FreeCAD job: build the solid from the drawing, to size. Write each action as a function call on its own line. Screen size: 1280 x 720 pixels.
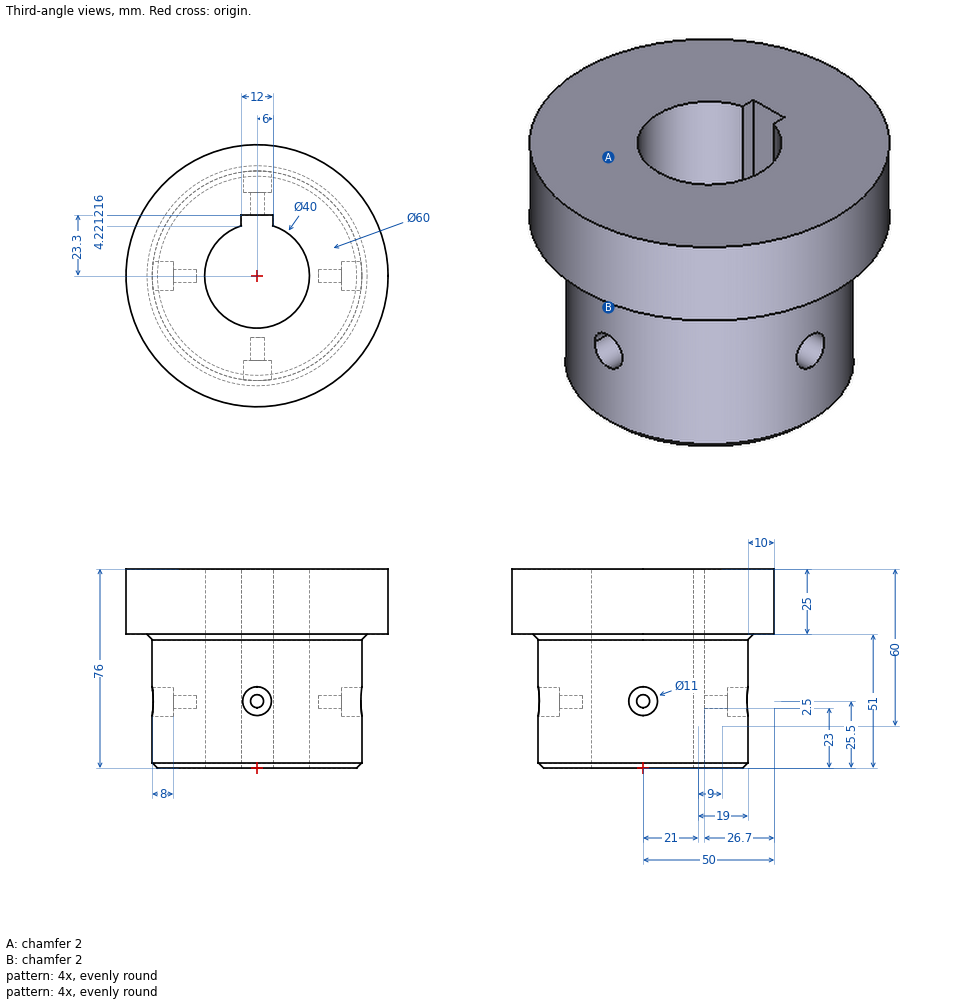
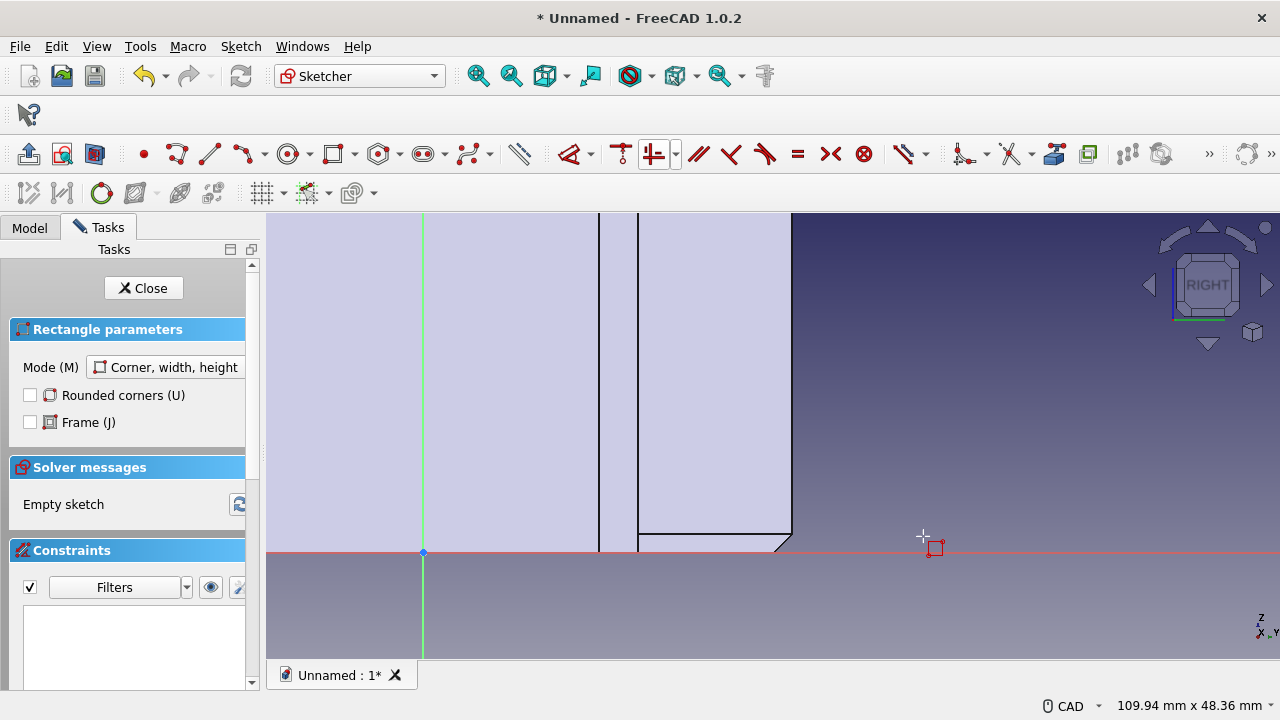
click(638, 318)
move(885, 341)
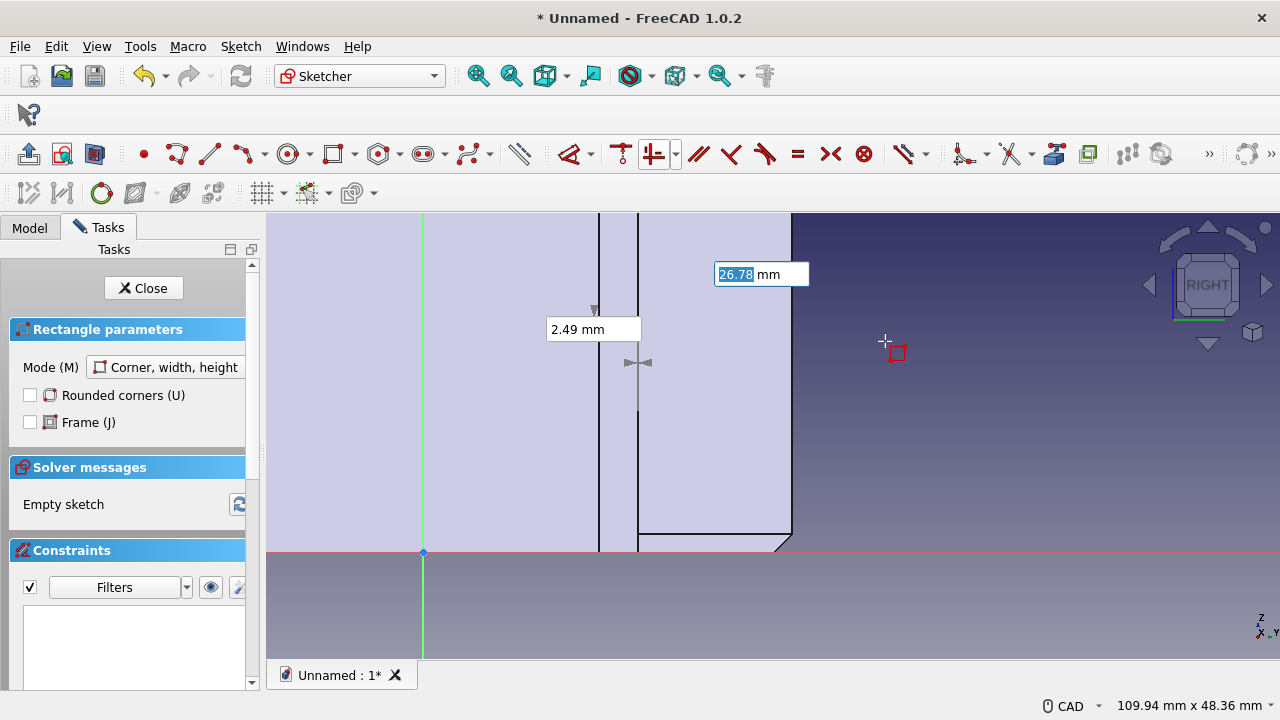
text(26.7)
key(Tab)
text(2.5)
key(Return)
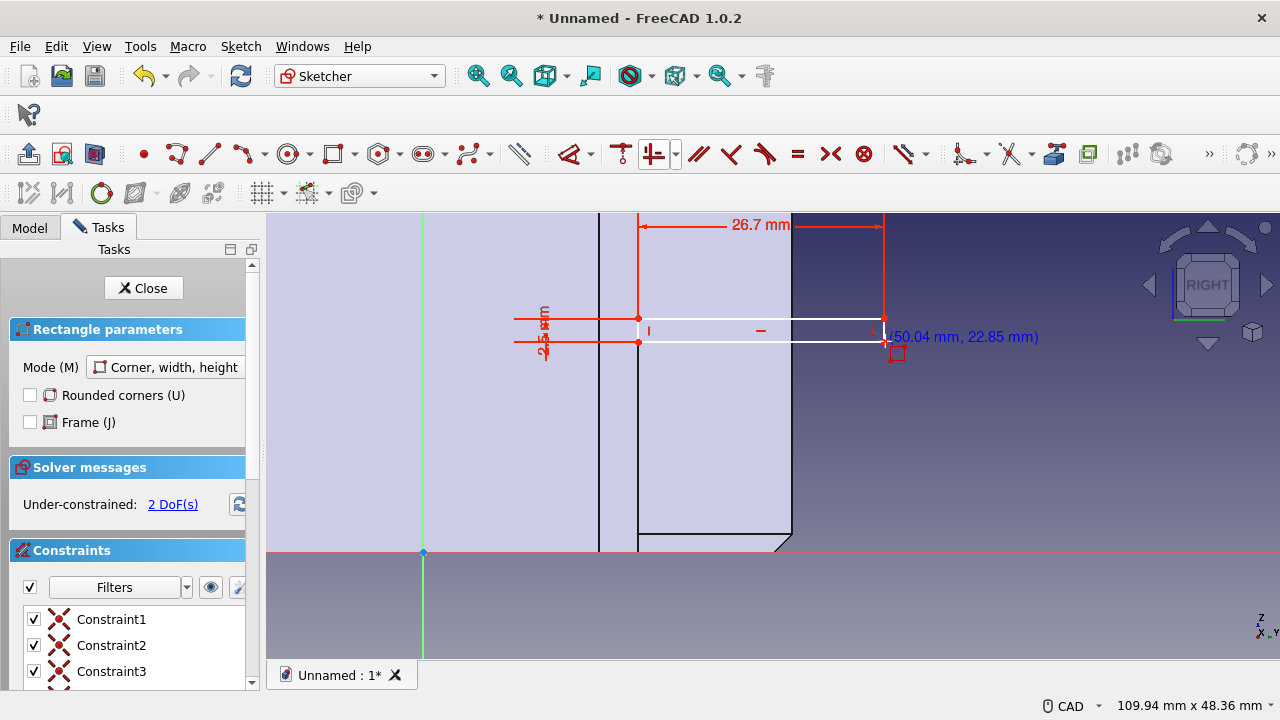
key(g)
key(l)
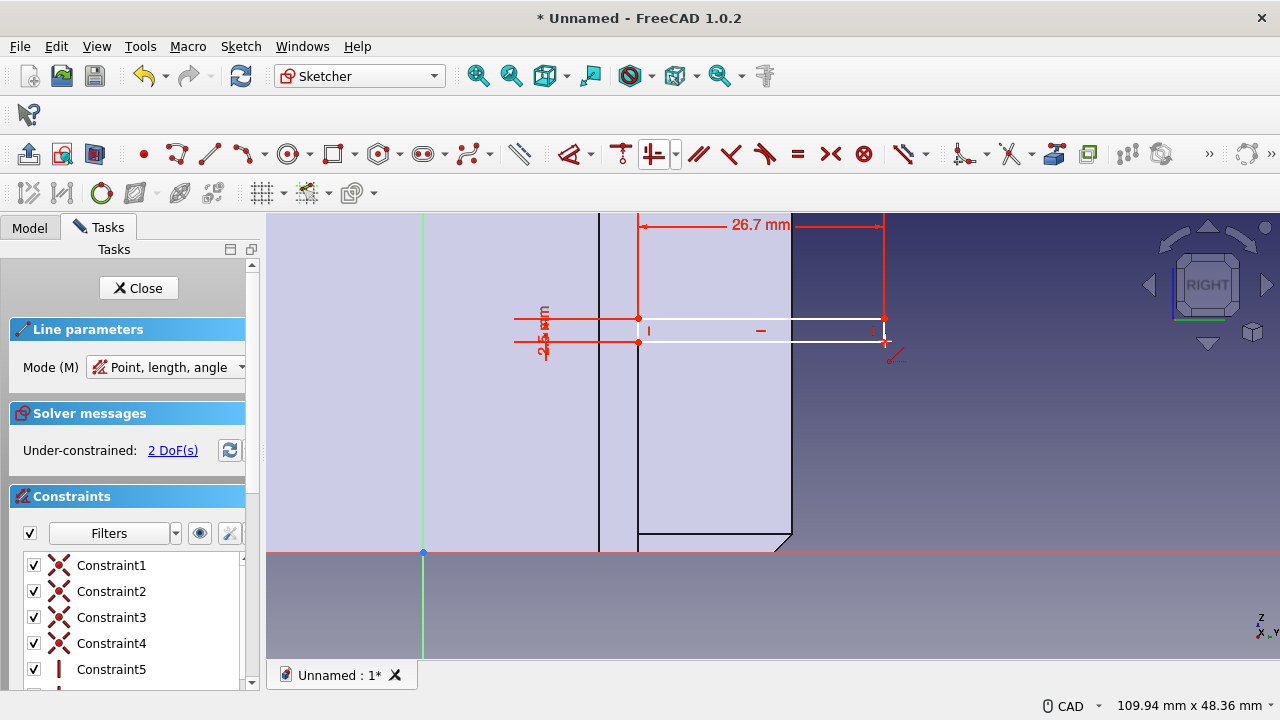
click(909, 318)
click(983, 318)
key(Escape)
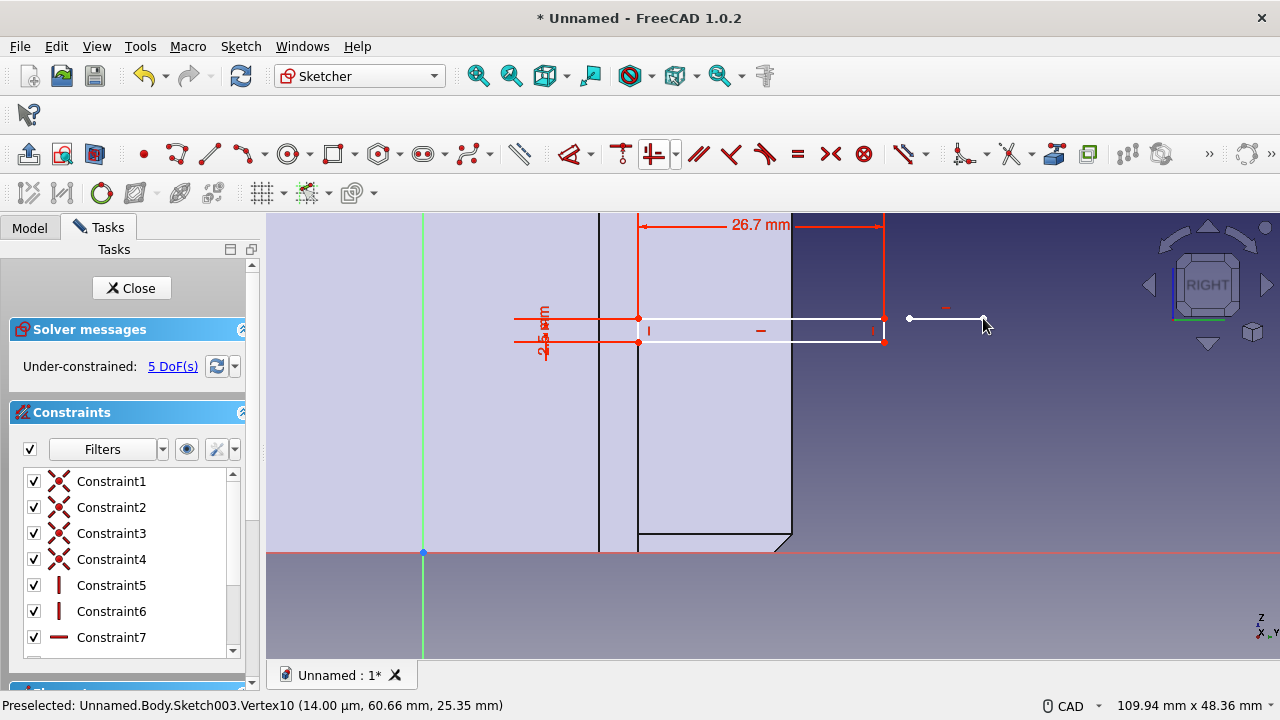
click(931, 319)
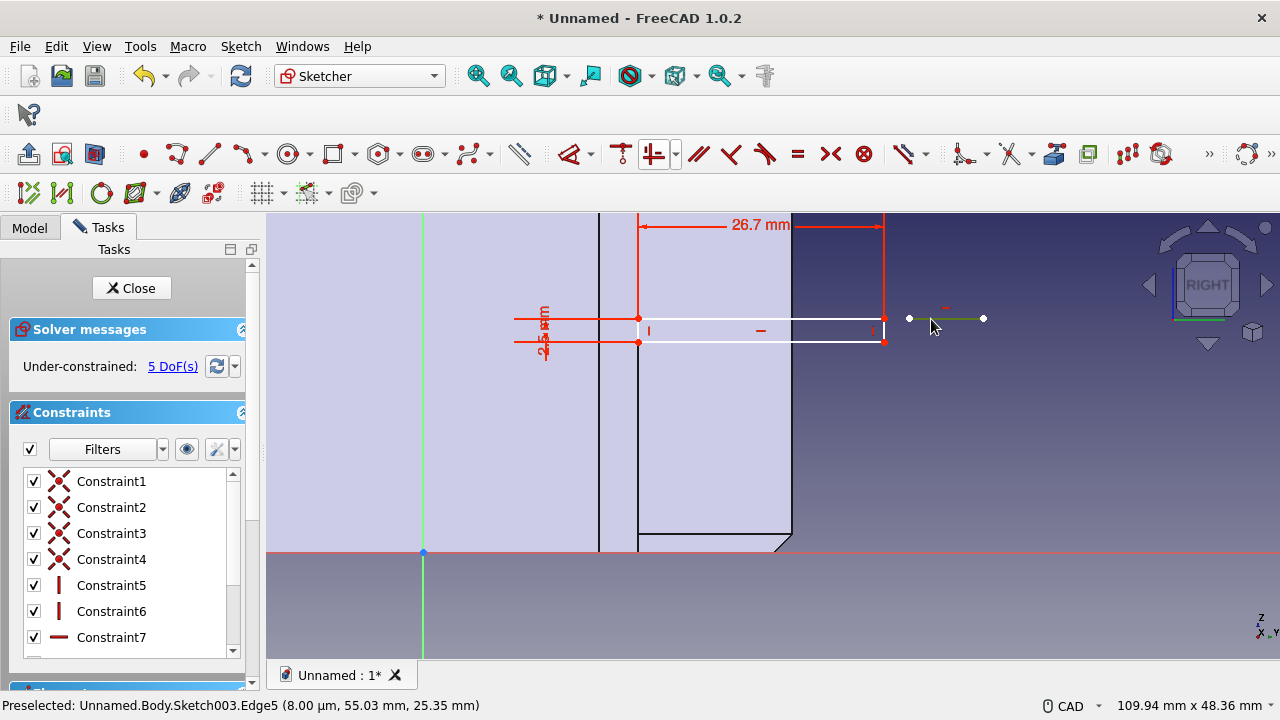
click(520, 154)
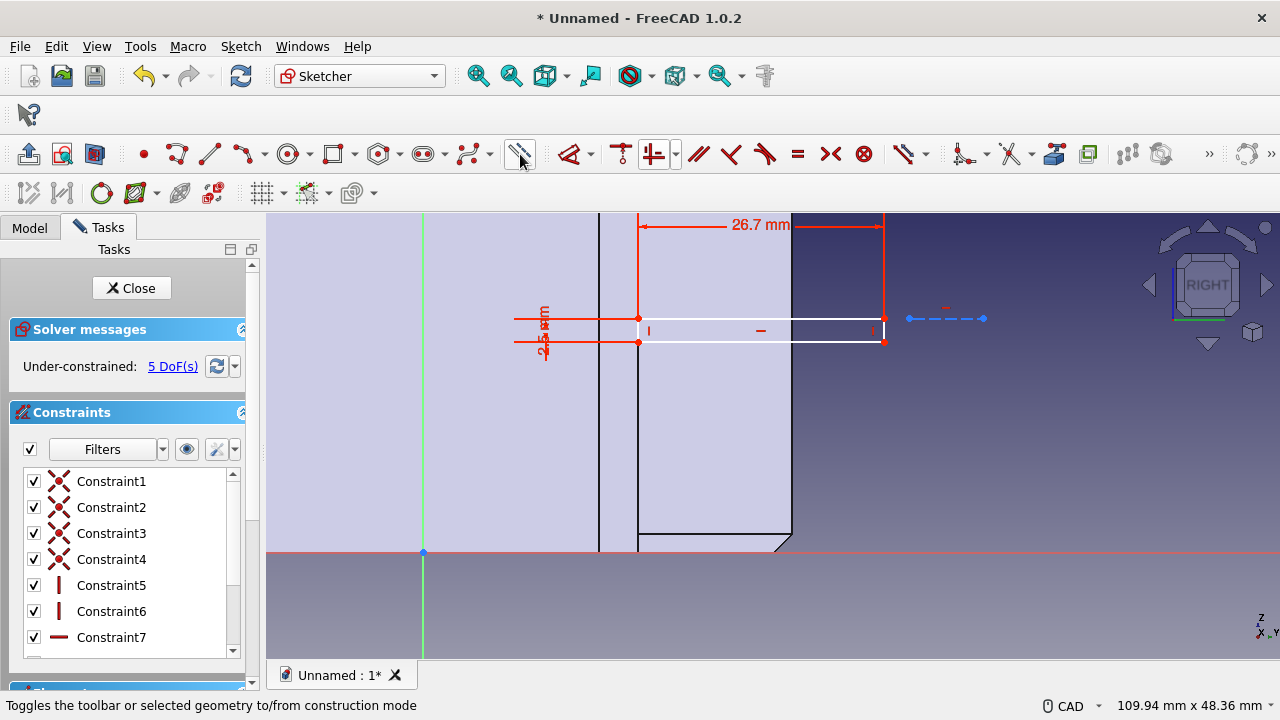
key(d)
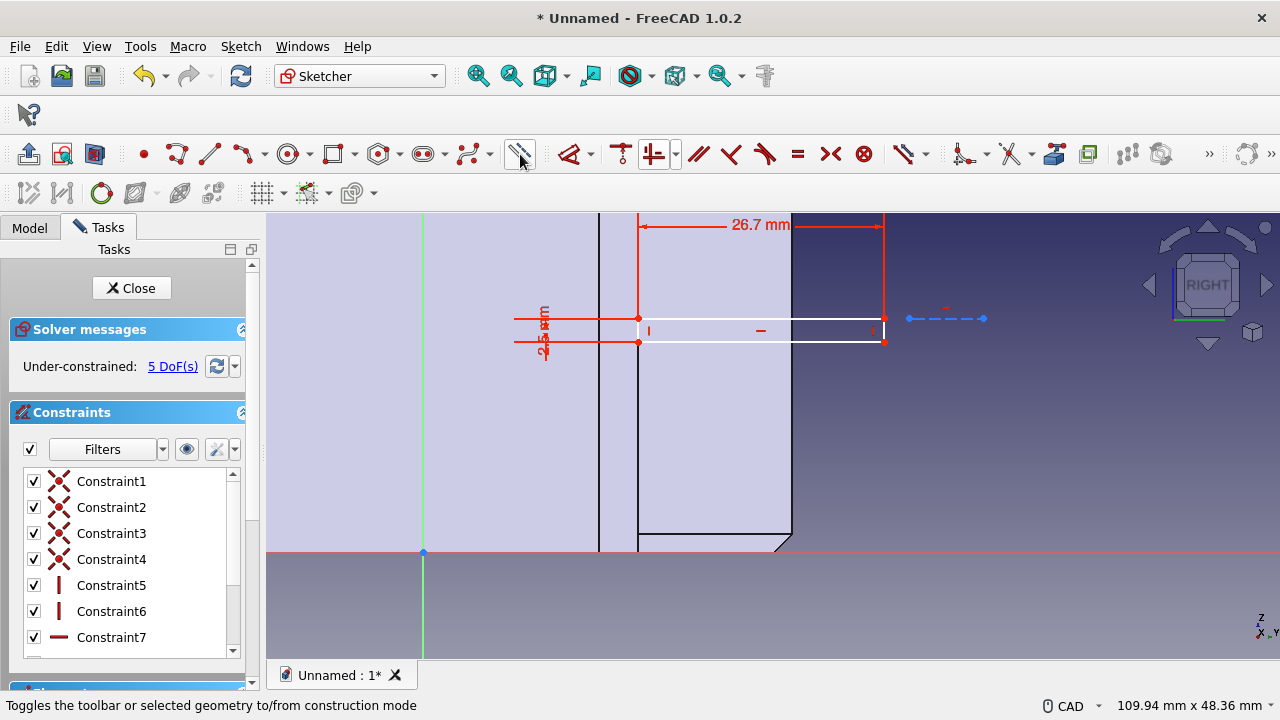
click(638, 342)
click(389, 447)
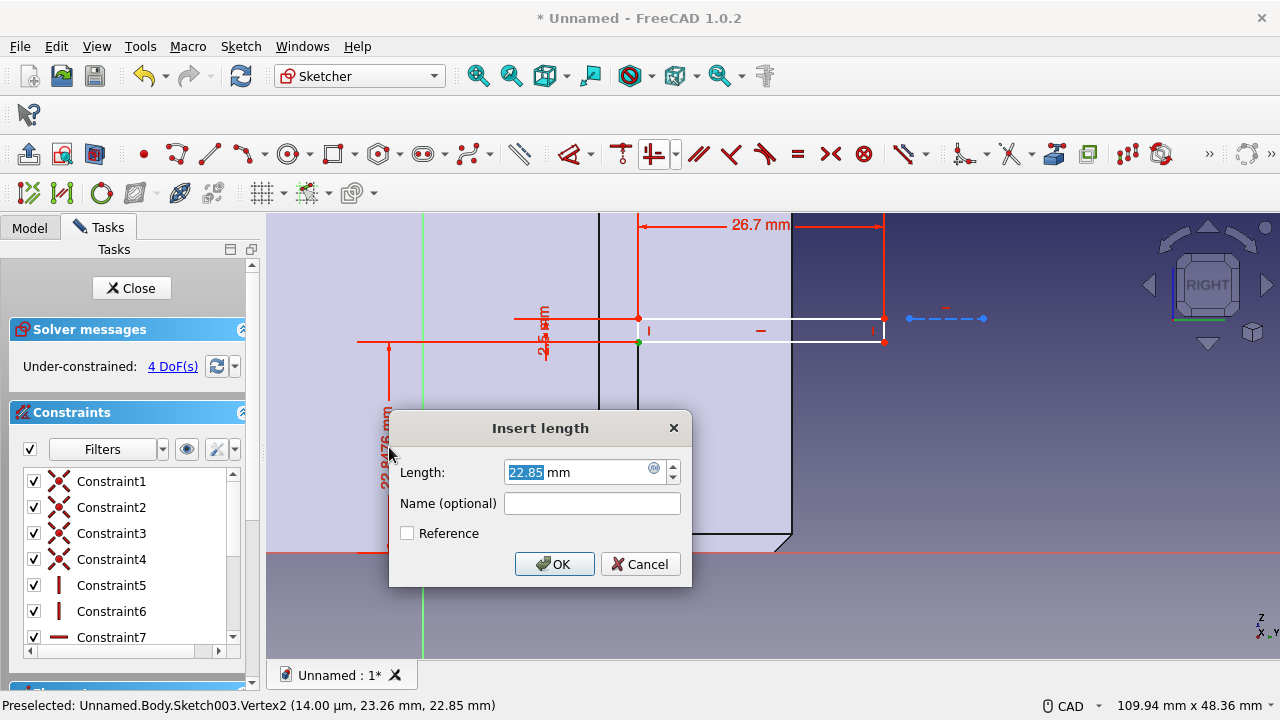
text(23)
key(Return)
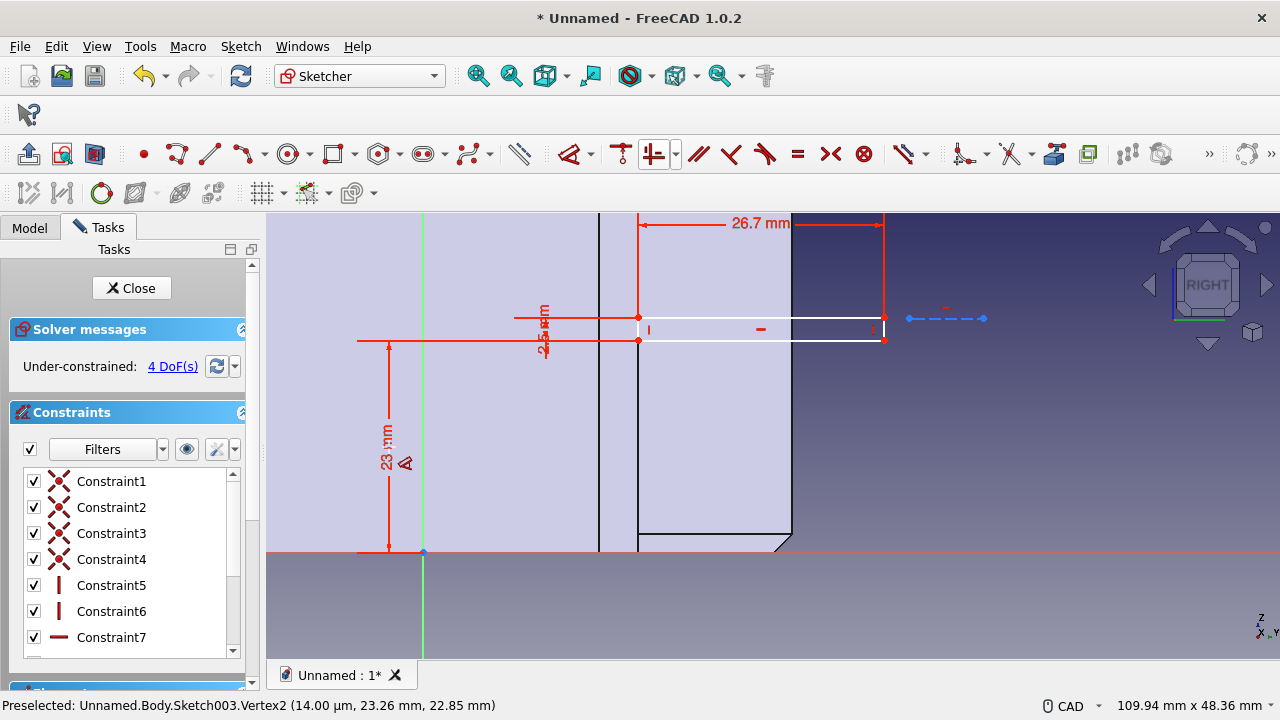
click(884, 341)
click(654, 587)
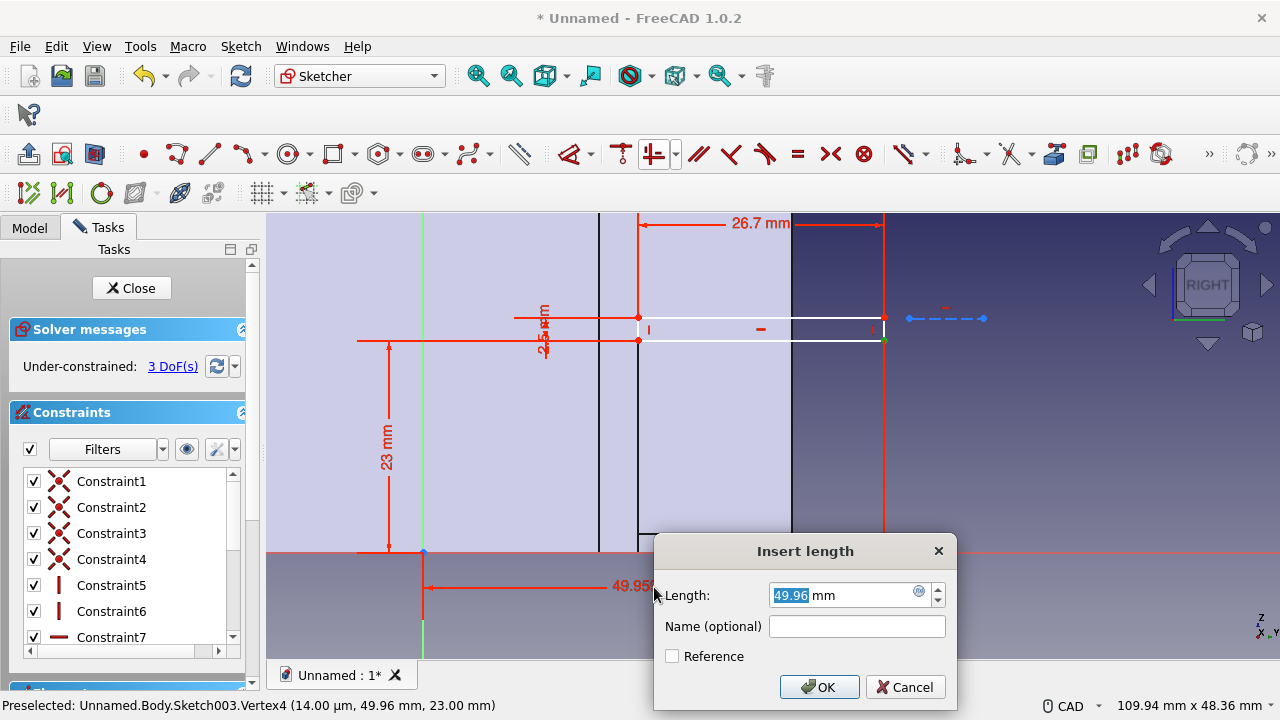
text(50)
key(Return)